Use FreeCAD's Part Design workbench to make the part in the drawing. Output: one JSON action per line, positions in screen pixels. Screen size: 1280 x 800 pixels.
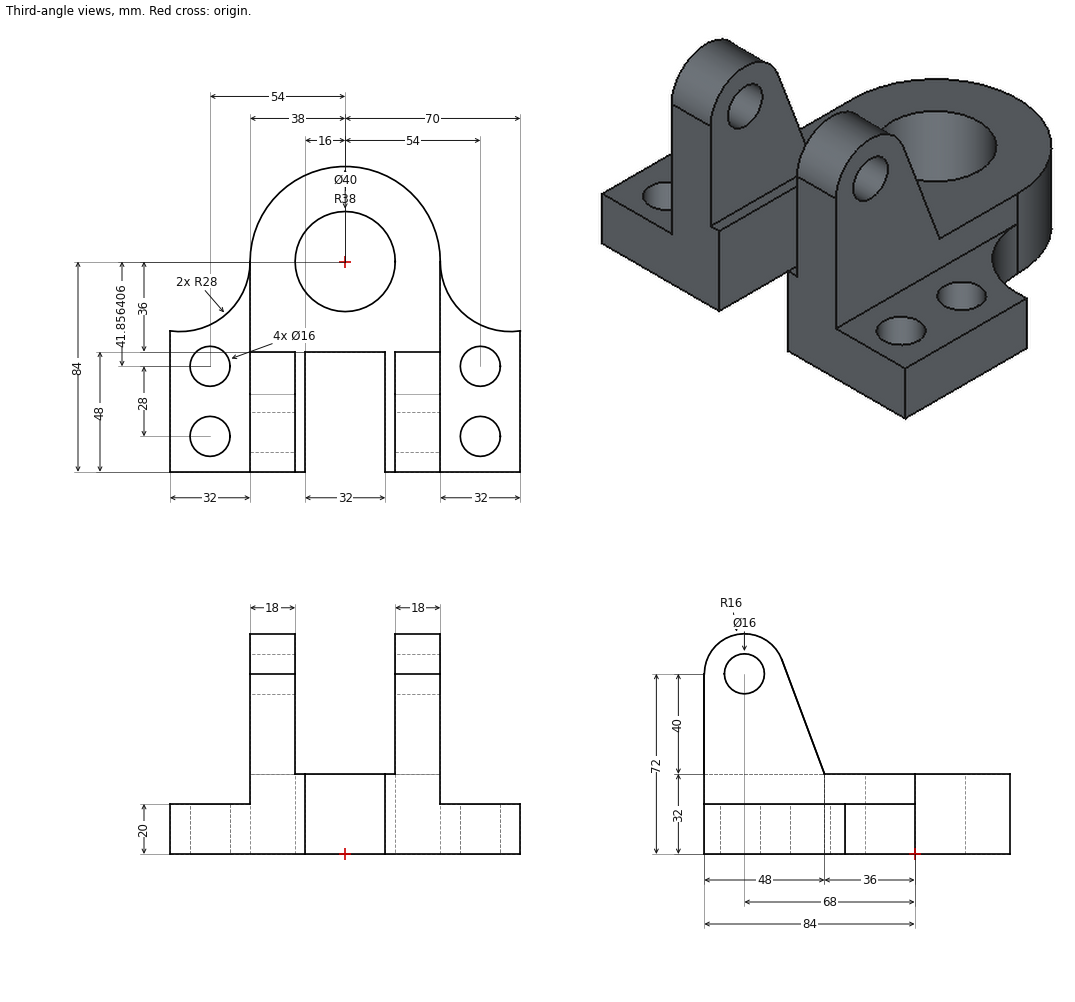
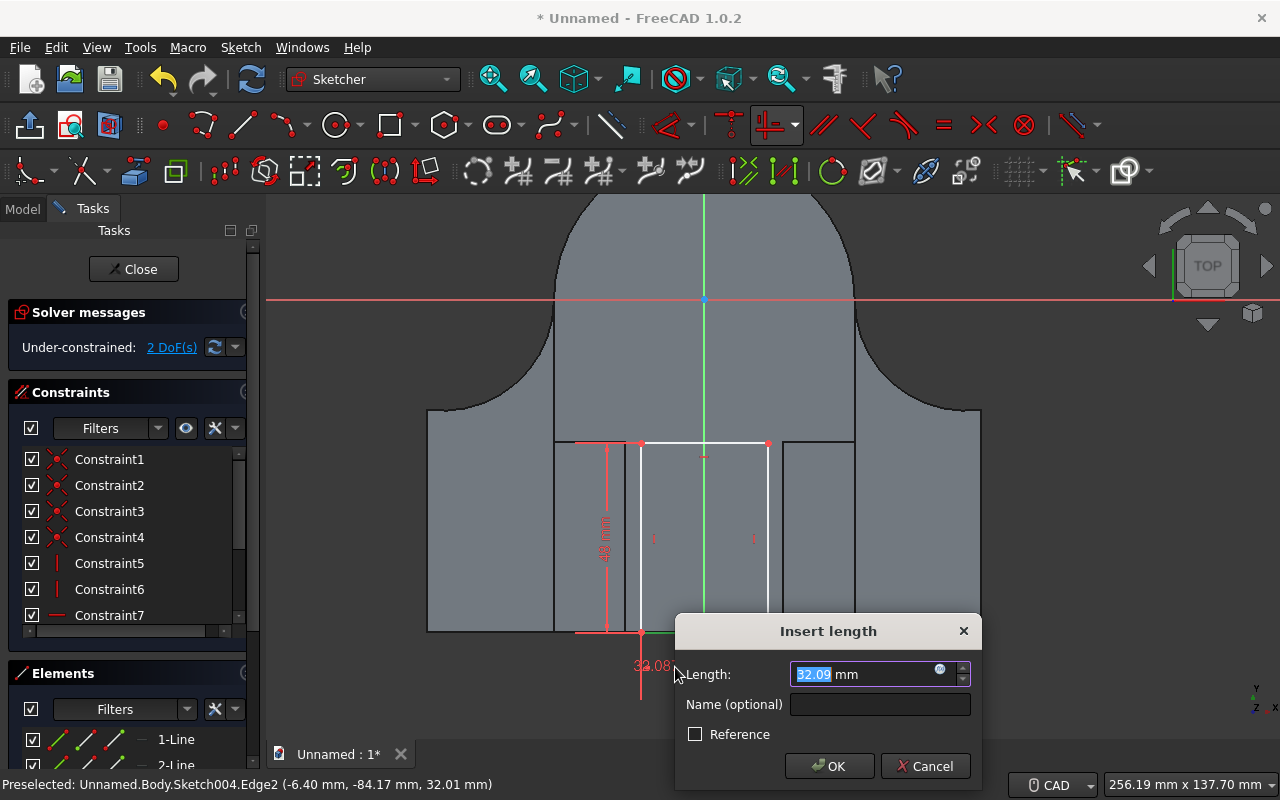
{"action": "type", "text": "32"}
{"action": "key", "text": "Return"}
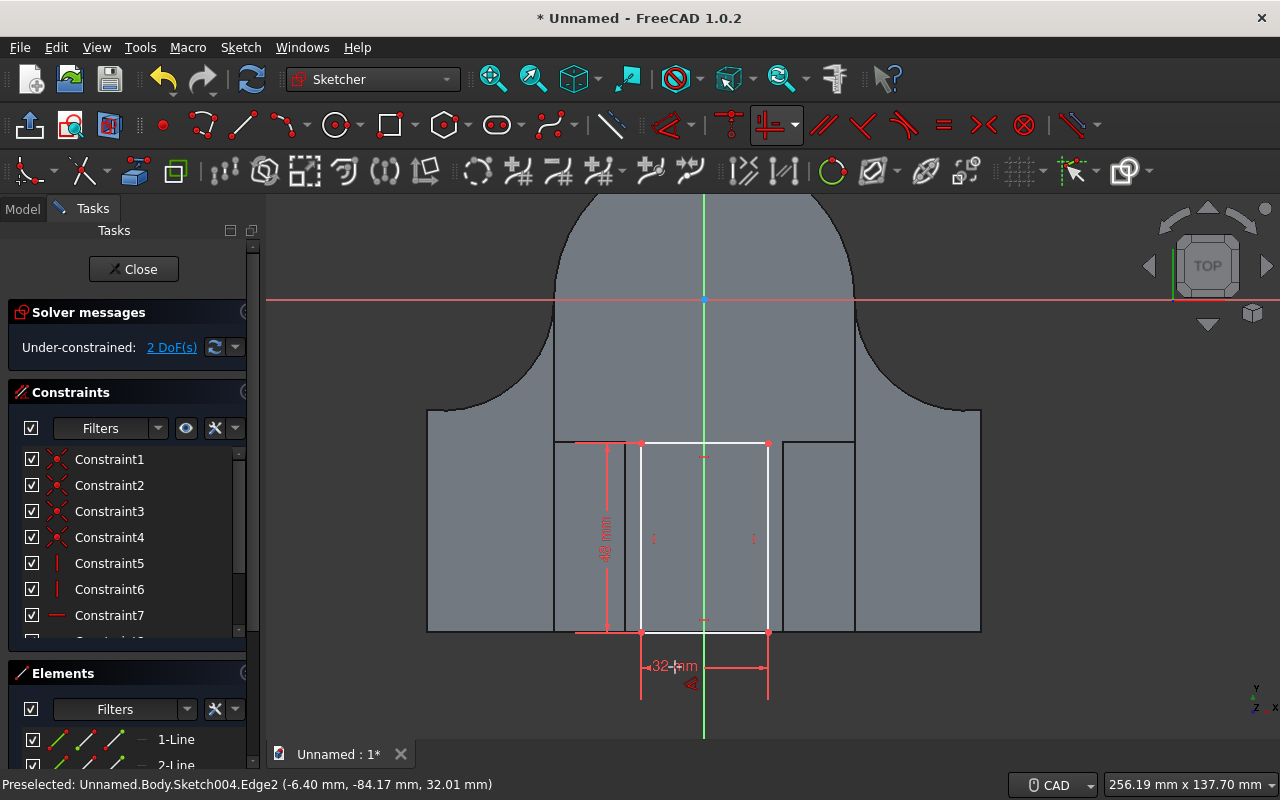
{"action": "left_click", "coordinate": [641, 443]}
{"action": "left_click", "coordinate": [673, 266]}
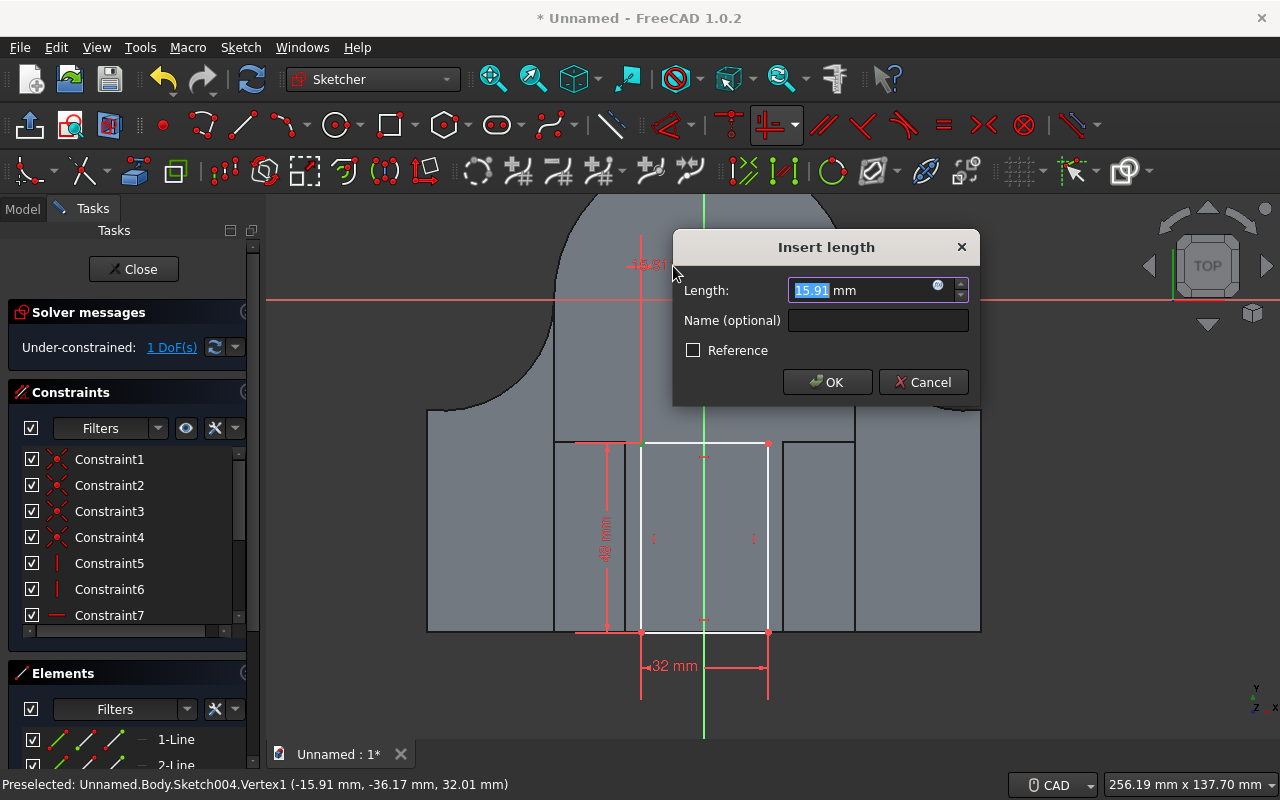
{"action": "type", "text": "16"}
{"action": "key", "text": "Return"}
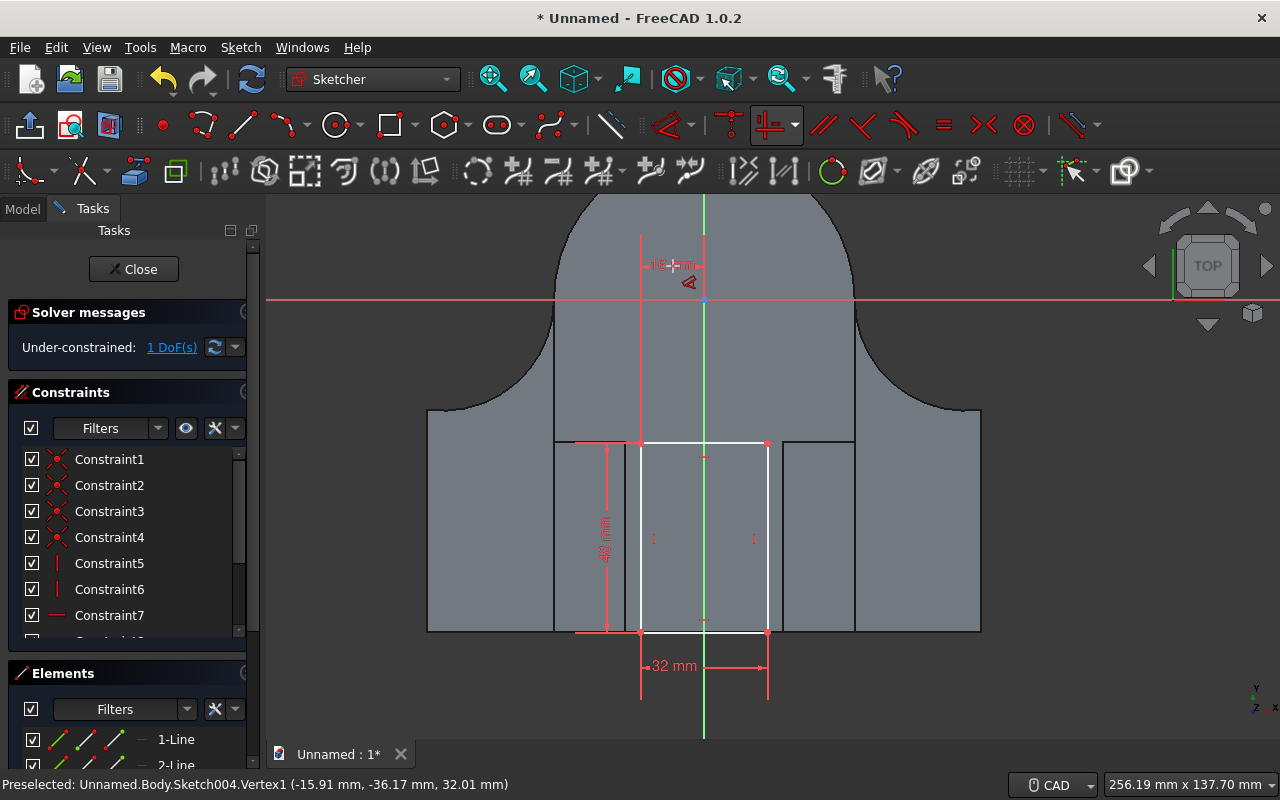
{"action": "left_click", "coordinate": [641, 443]}
{"action": "left_click", "coordinate": [607, 371]}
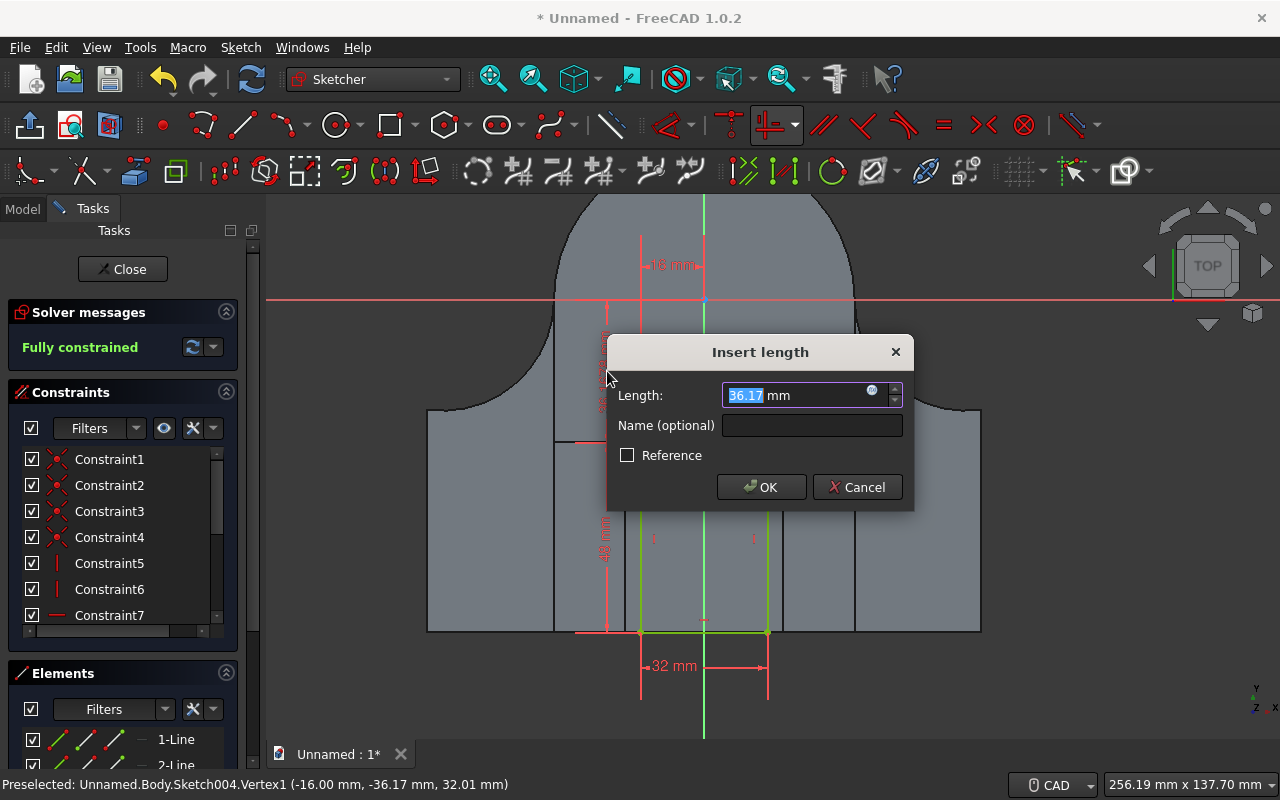
{"action": "type", "text": "36"}
{"action": "key", "text": "Return"}
{"action": "key", "text": "Escape"}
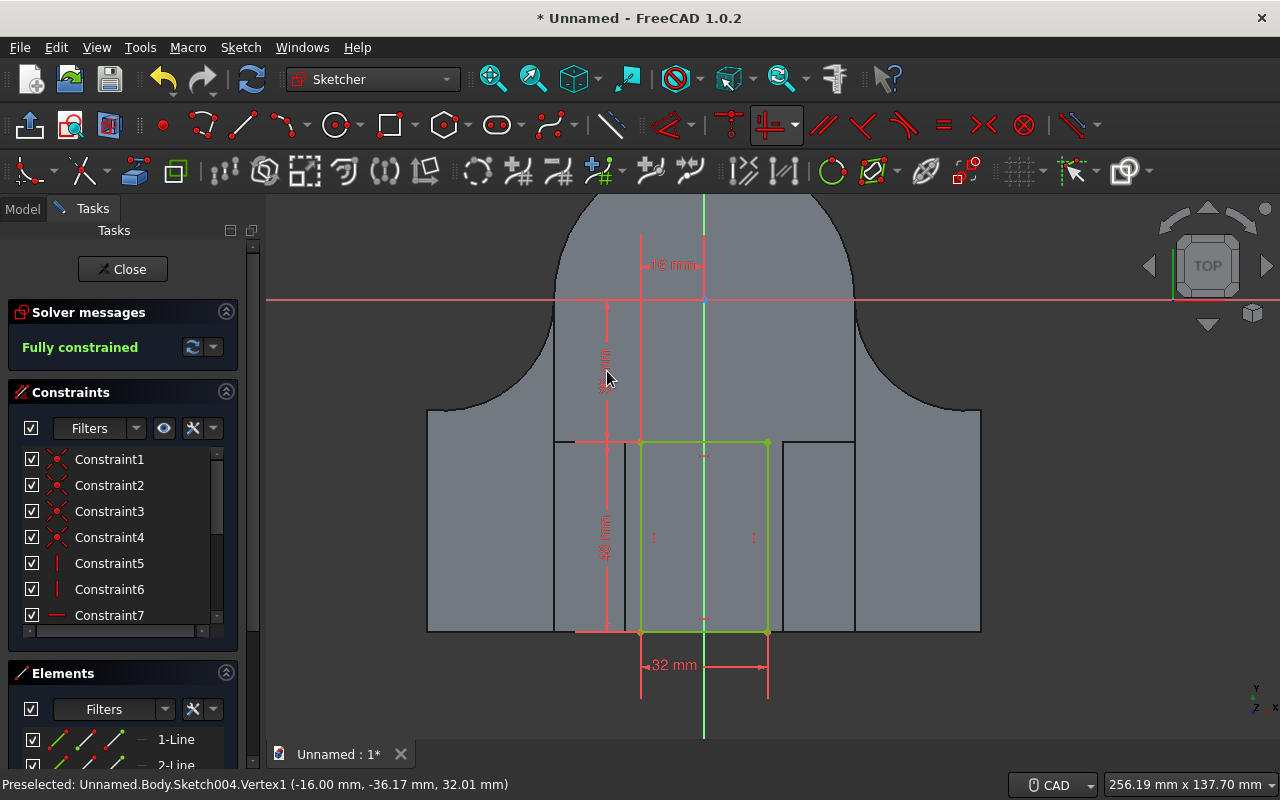
{"action": "left_click", "coordinate": [123, 269]}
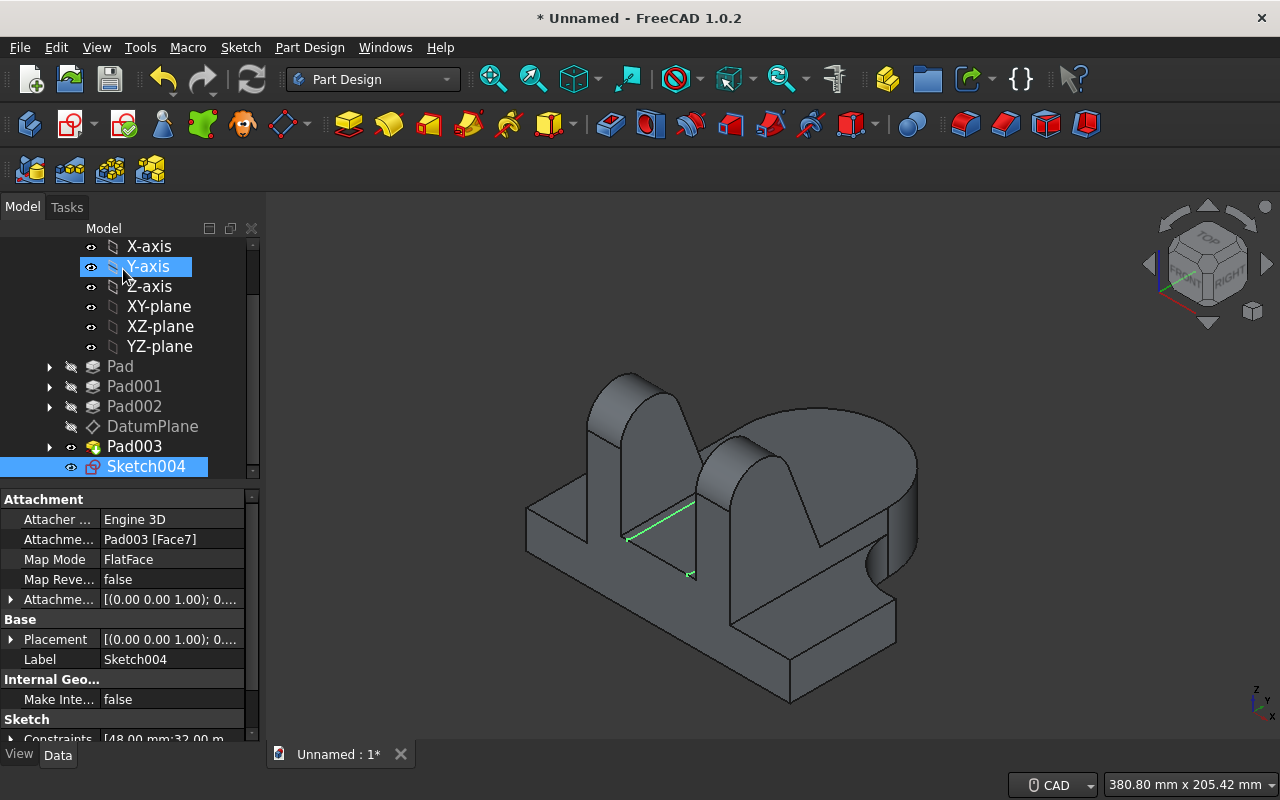
{"action": "left_click", "coordinate": [612, 124]}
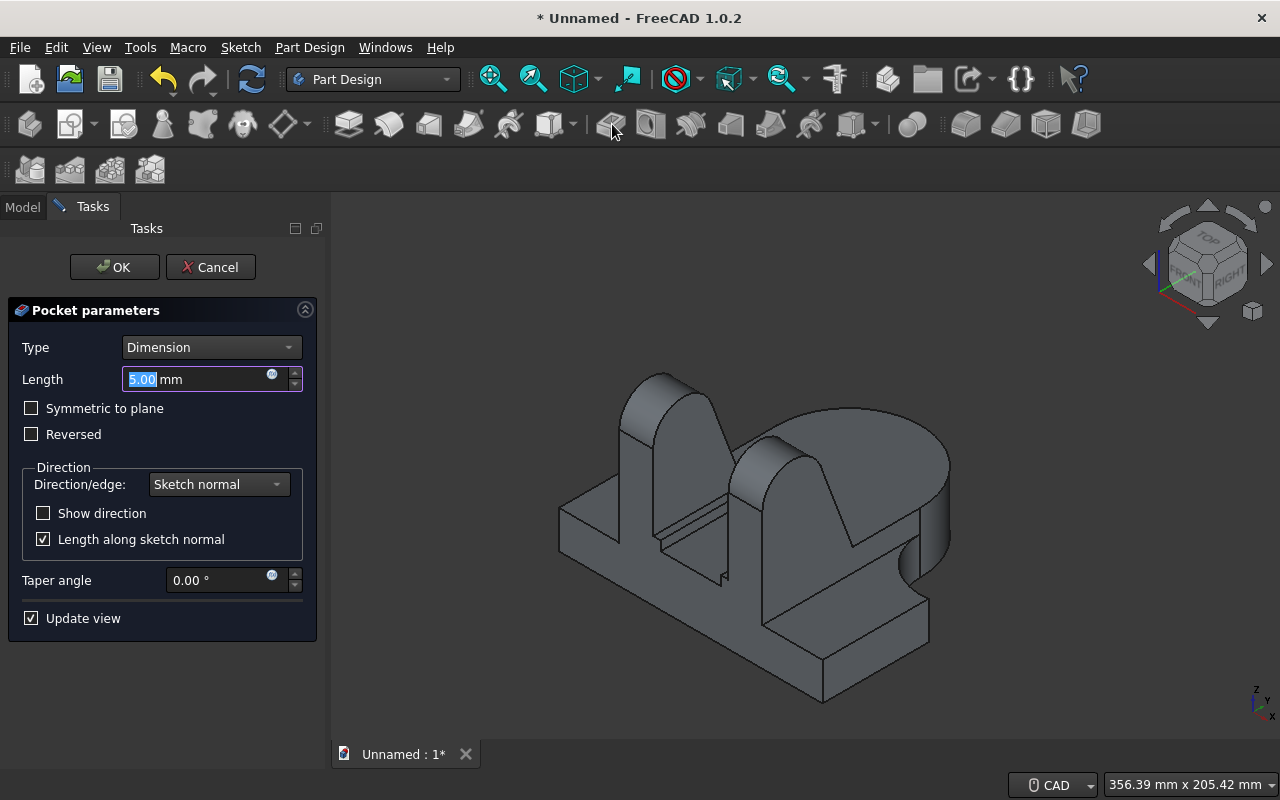
{"action": "left_click", "coordinate": [212, 348]}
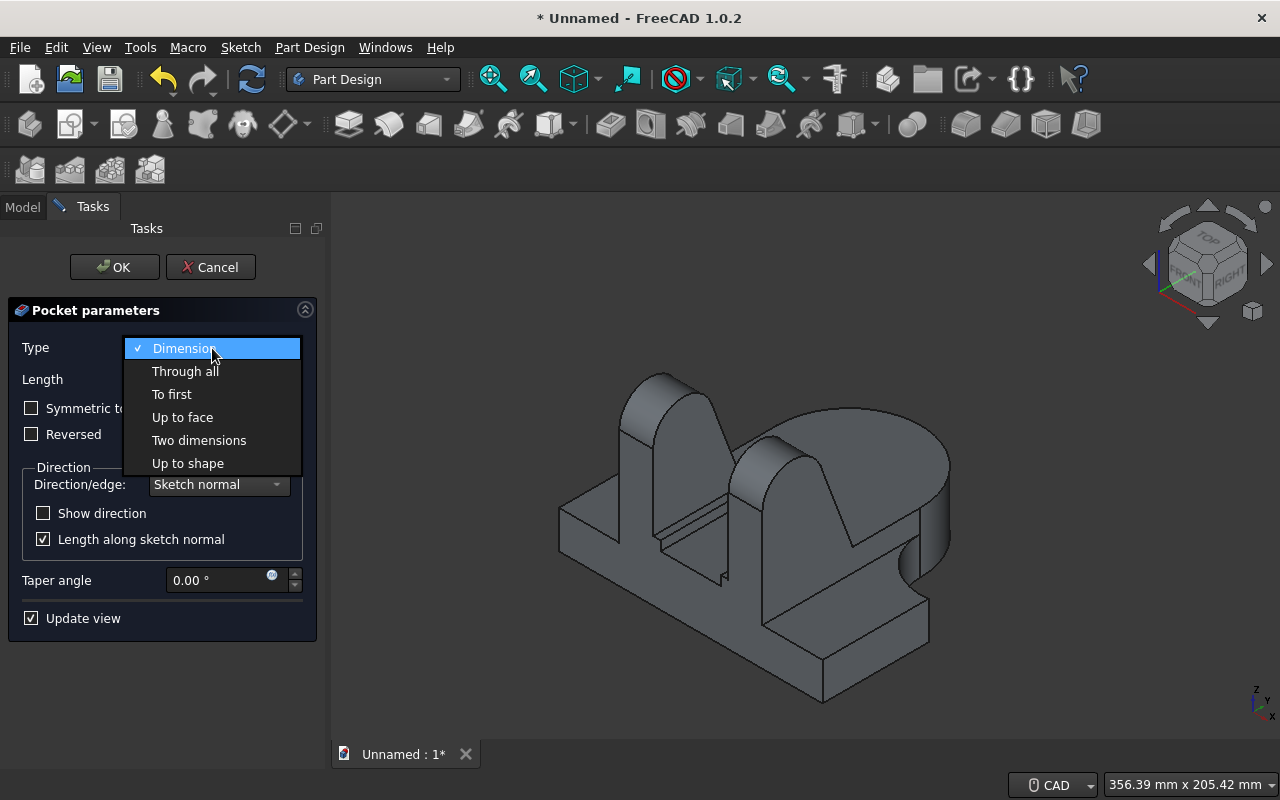
{"action": "left_click", "coordinate": [212, 372]}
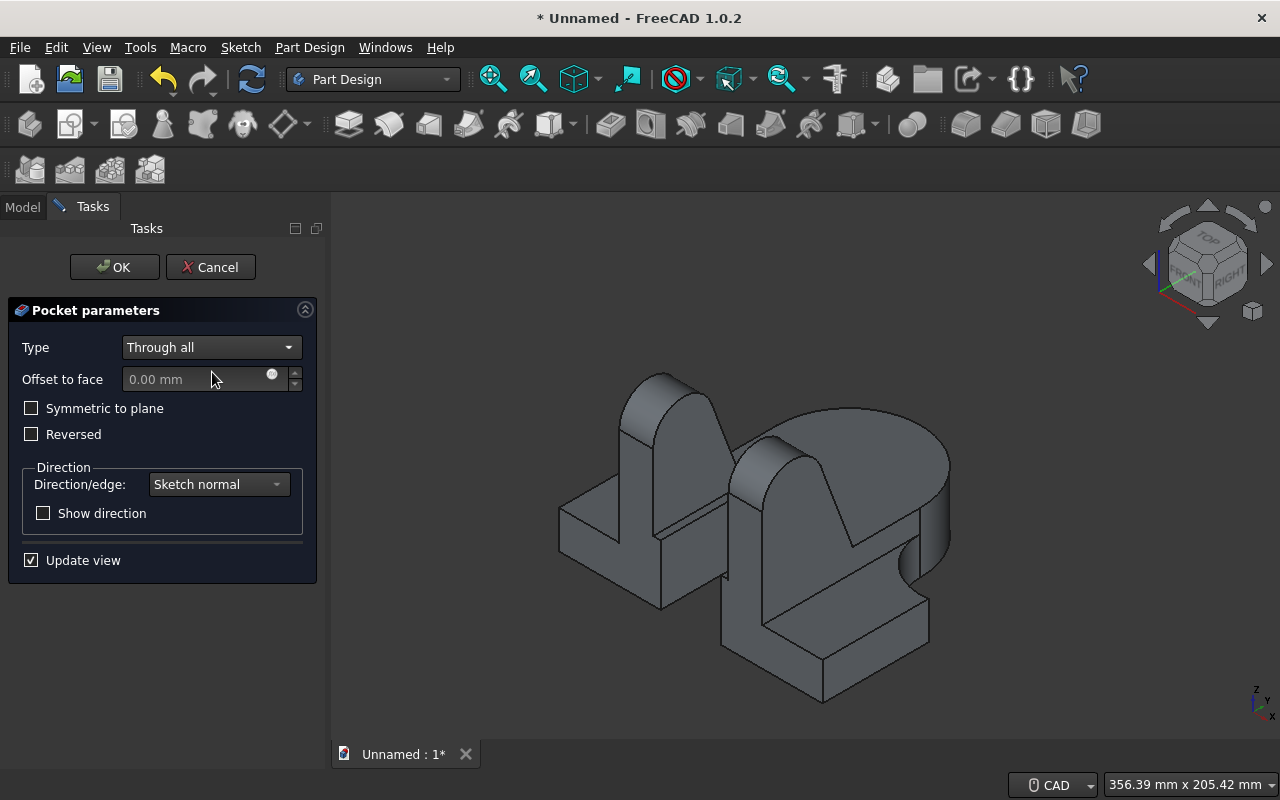
{"action": "left_click", "coordinate": [115, 267]}